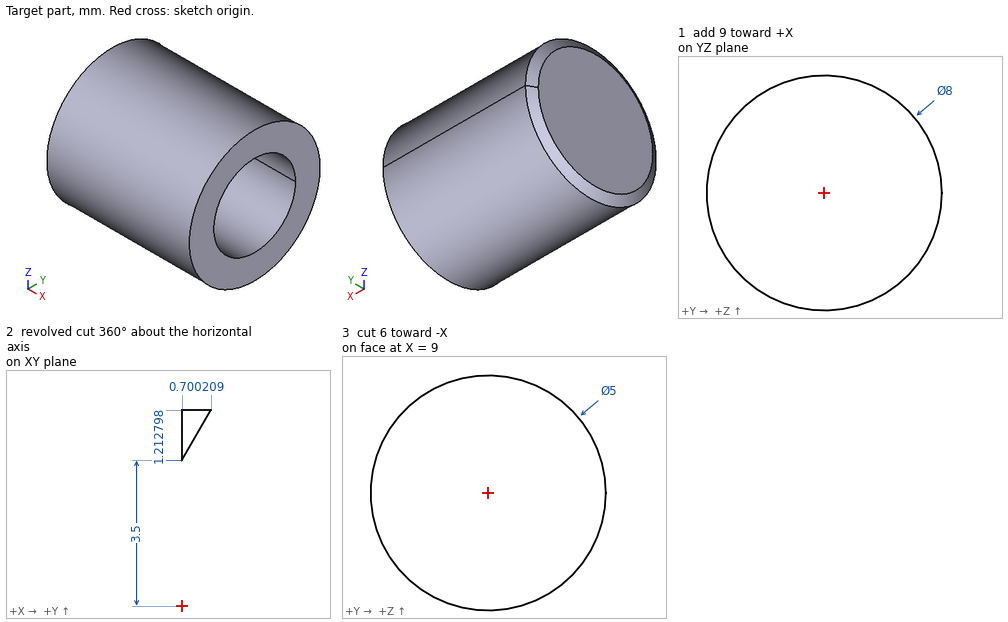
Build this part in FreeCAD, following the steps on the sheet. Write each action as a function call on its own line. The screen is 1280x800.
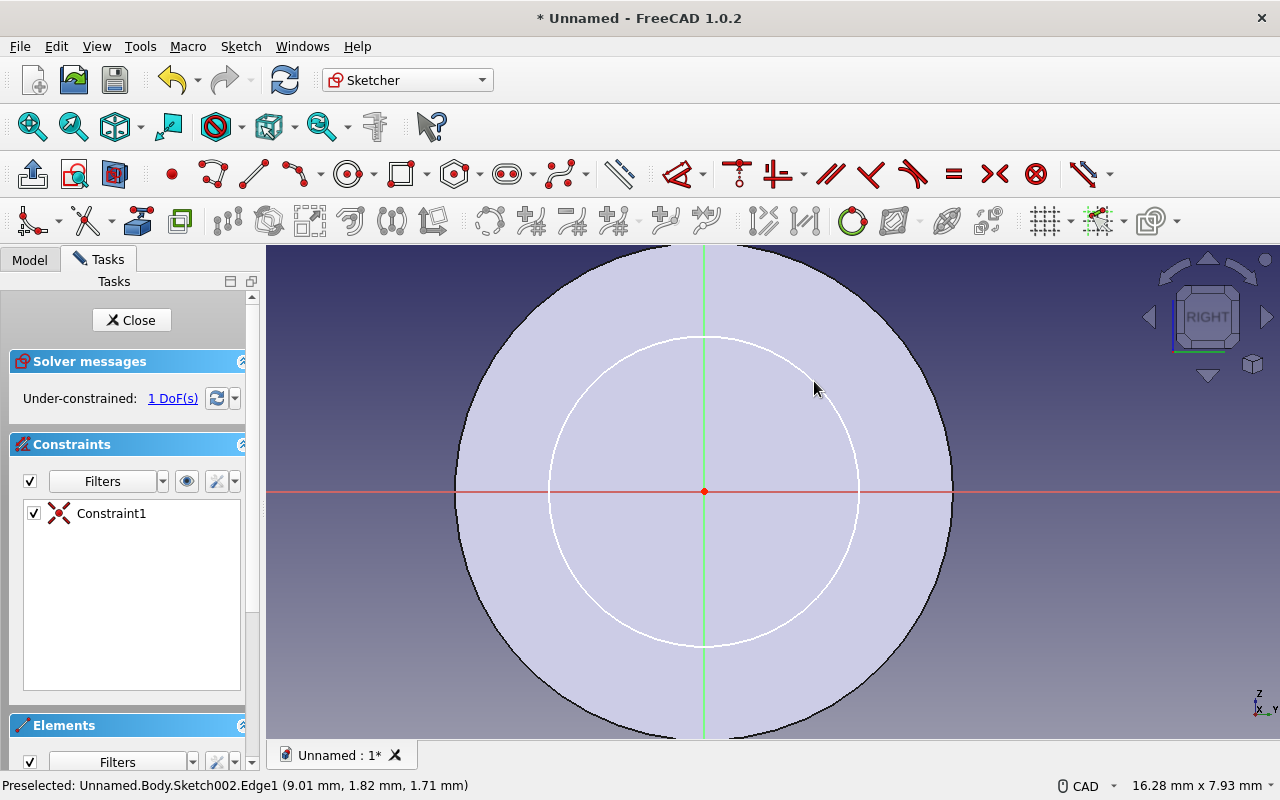
key(d)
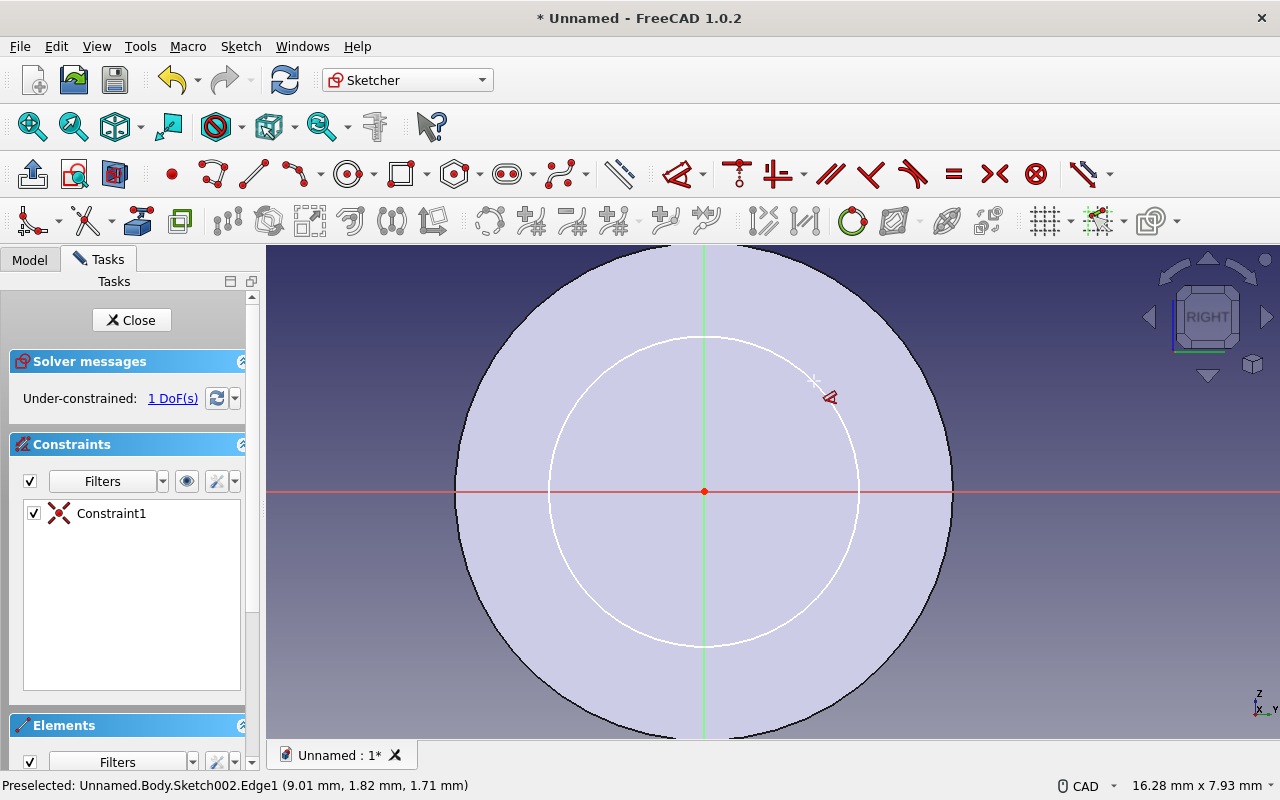
click(813, 381)
click(835, 358)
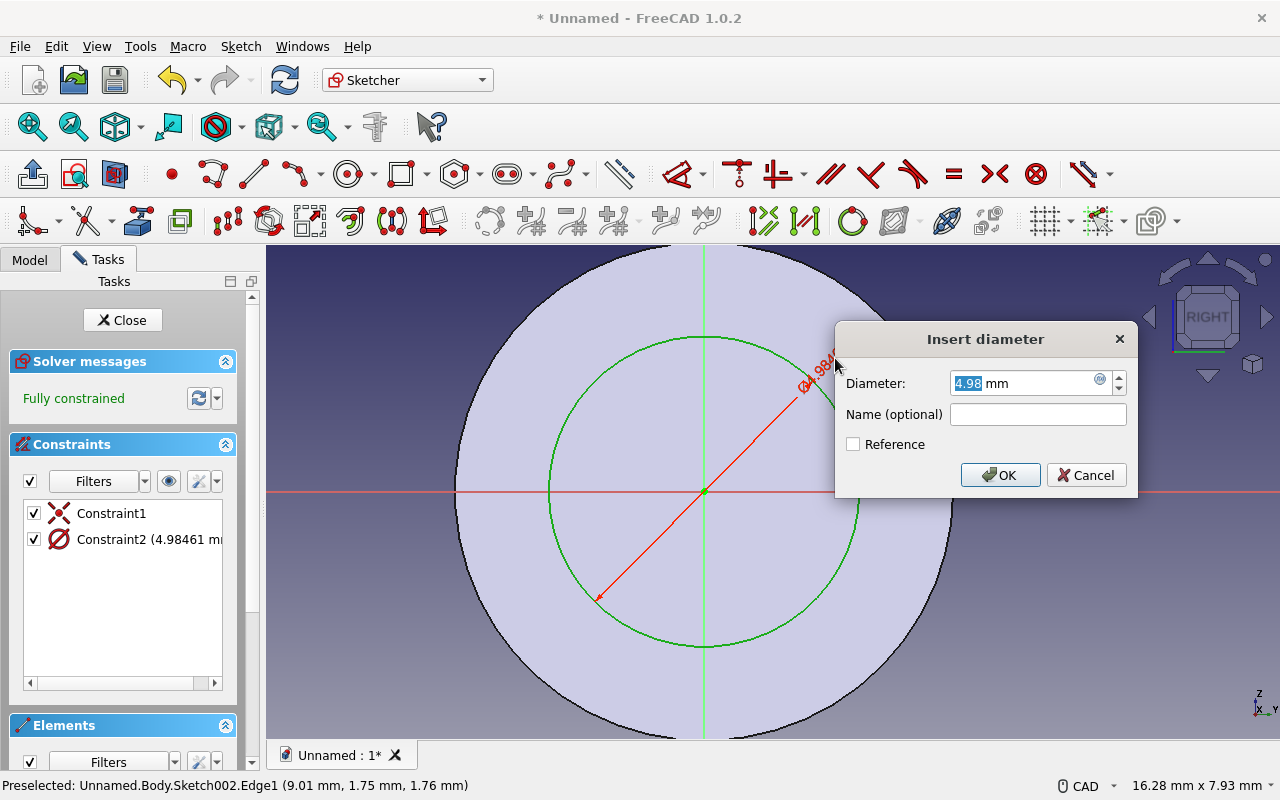
text(5)
key(Return)
key(Escape)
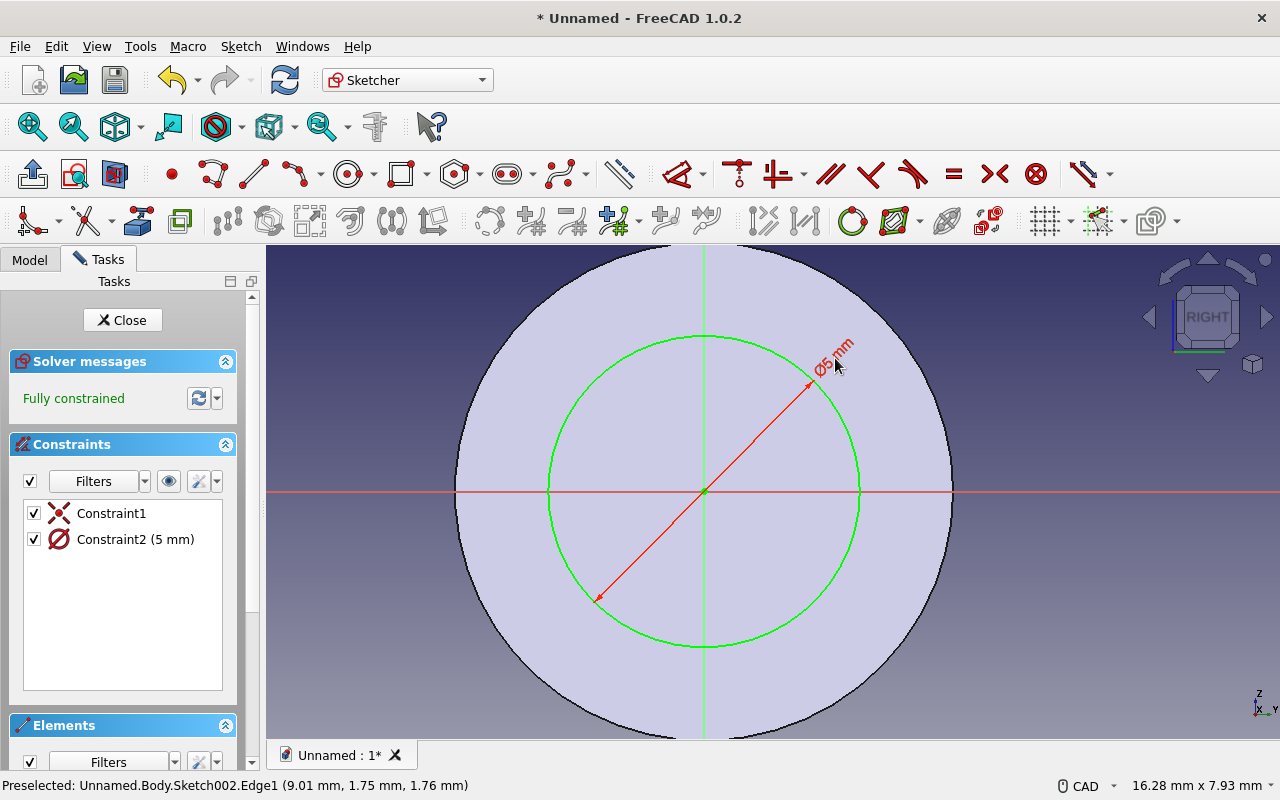
click(123, 320)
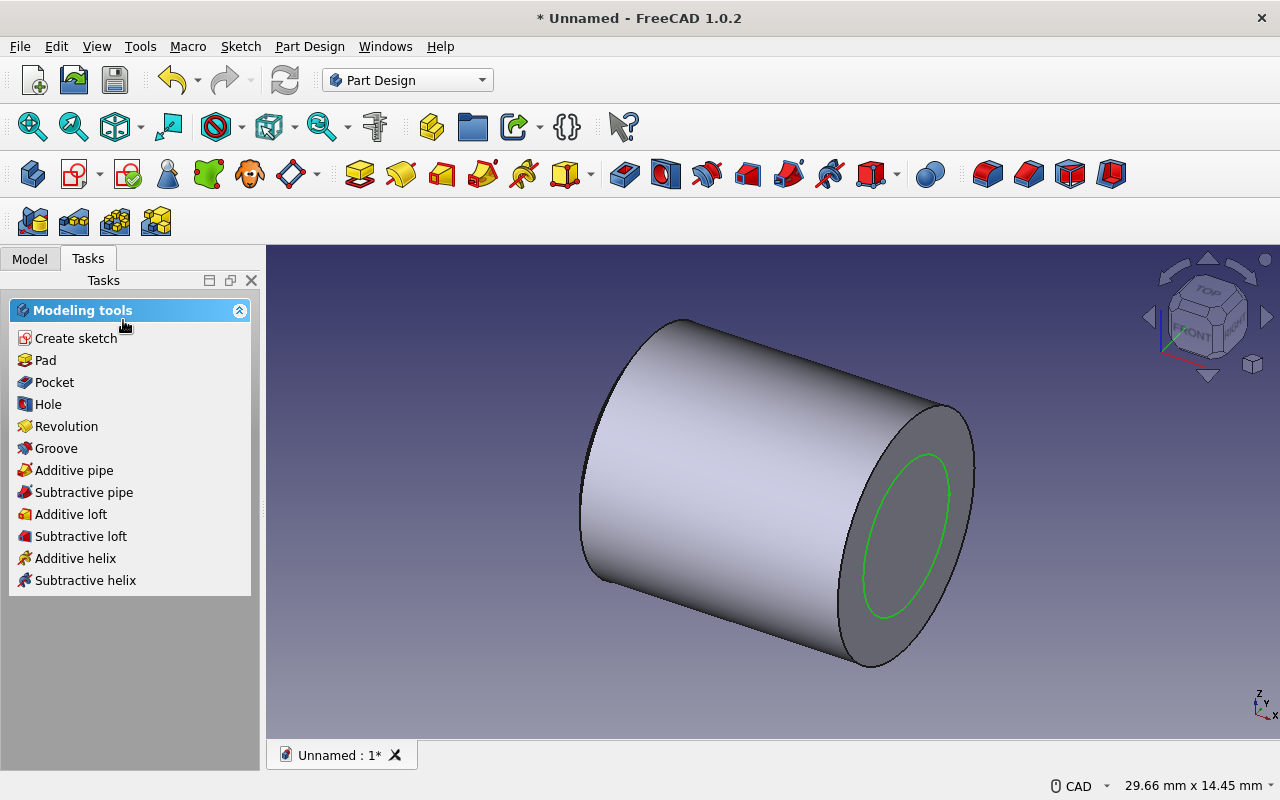
click(625, 174)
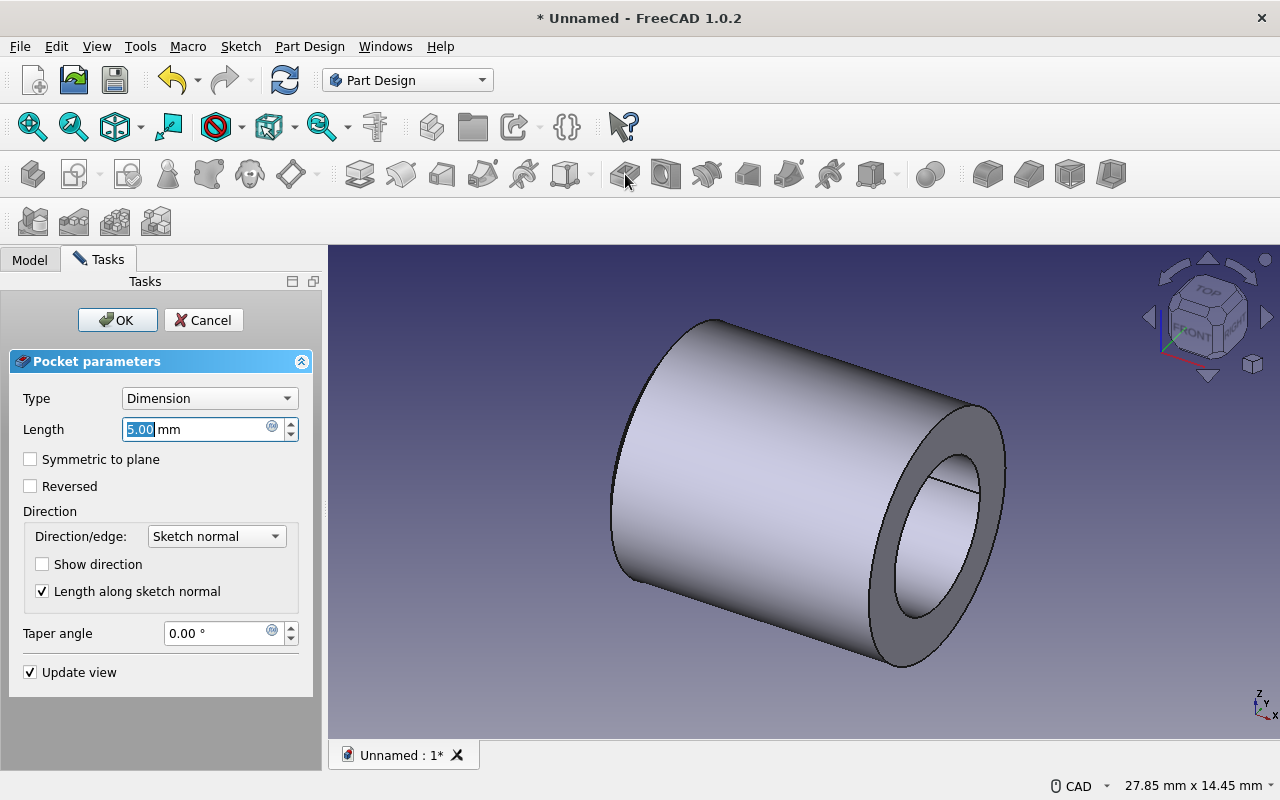
text(6)
key(Tab)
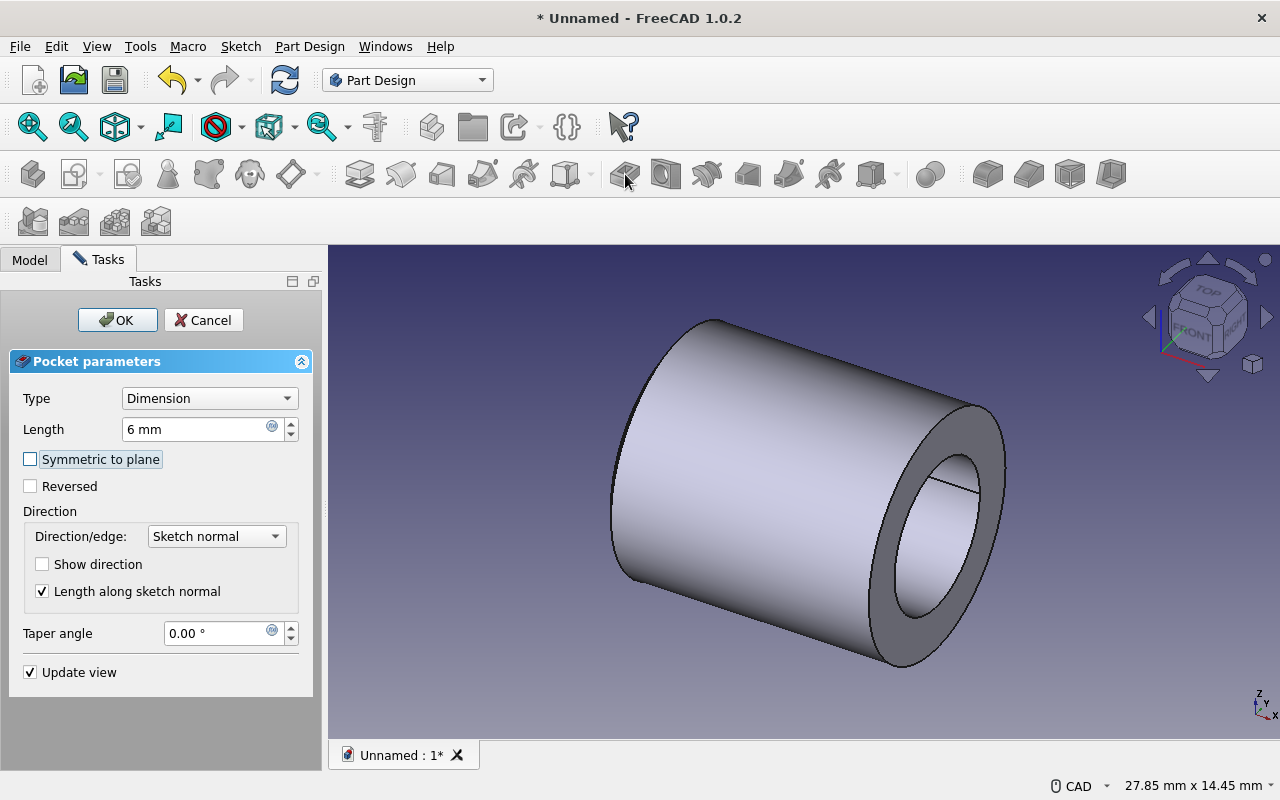
click(118, 320)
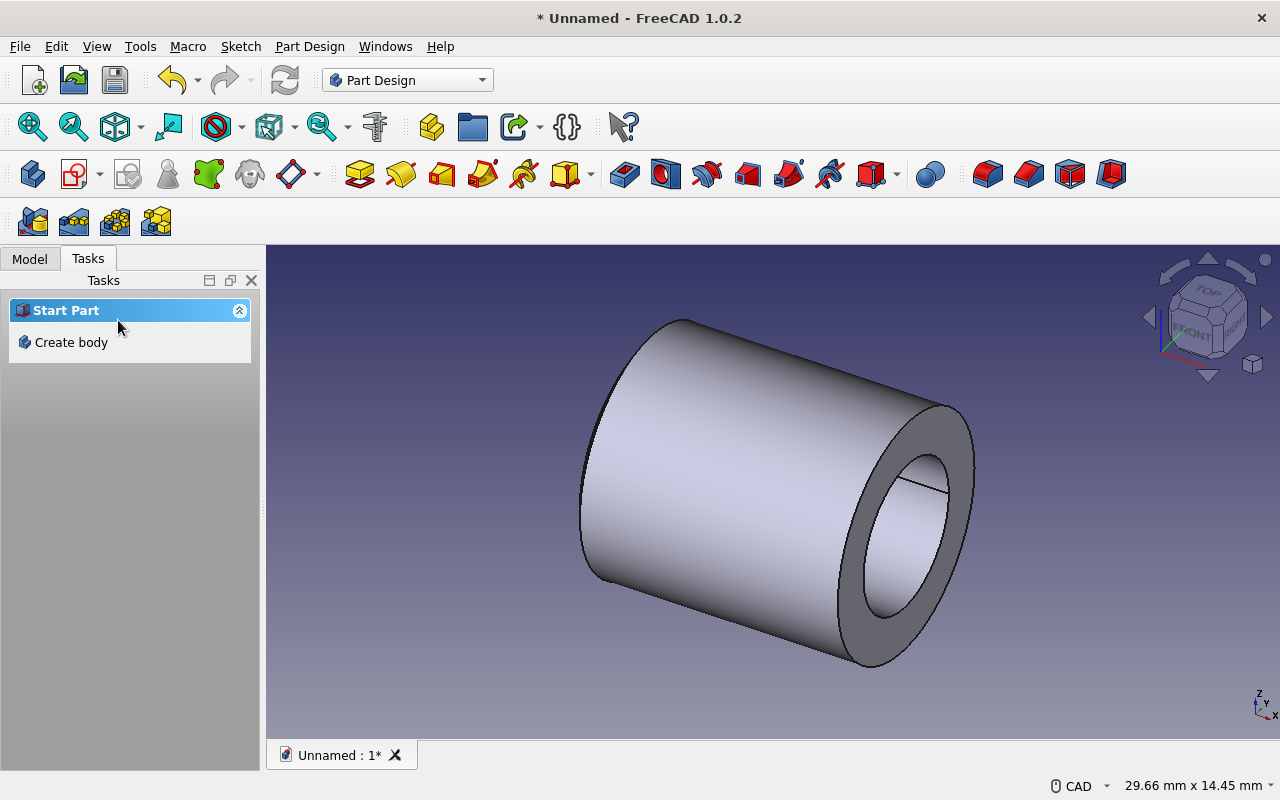
key(0)